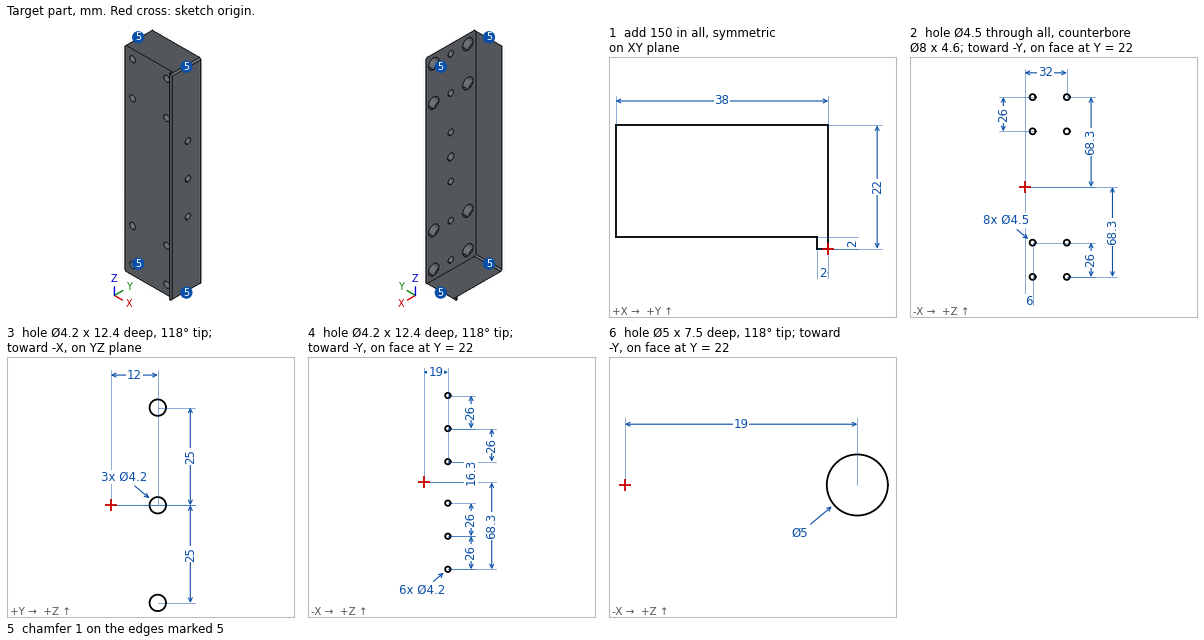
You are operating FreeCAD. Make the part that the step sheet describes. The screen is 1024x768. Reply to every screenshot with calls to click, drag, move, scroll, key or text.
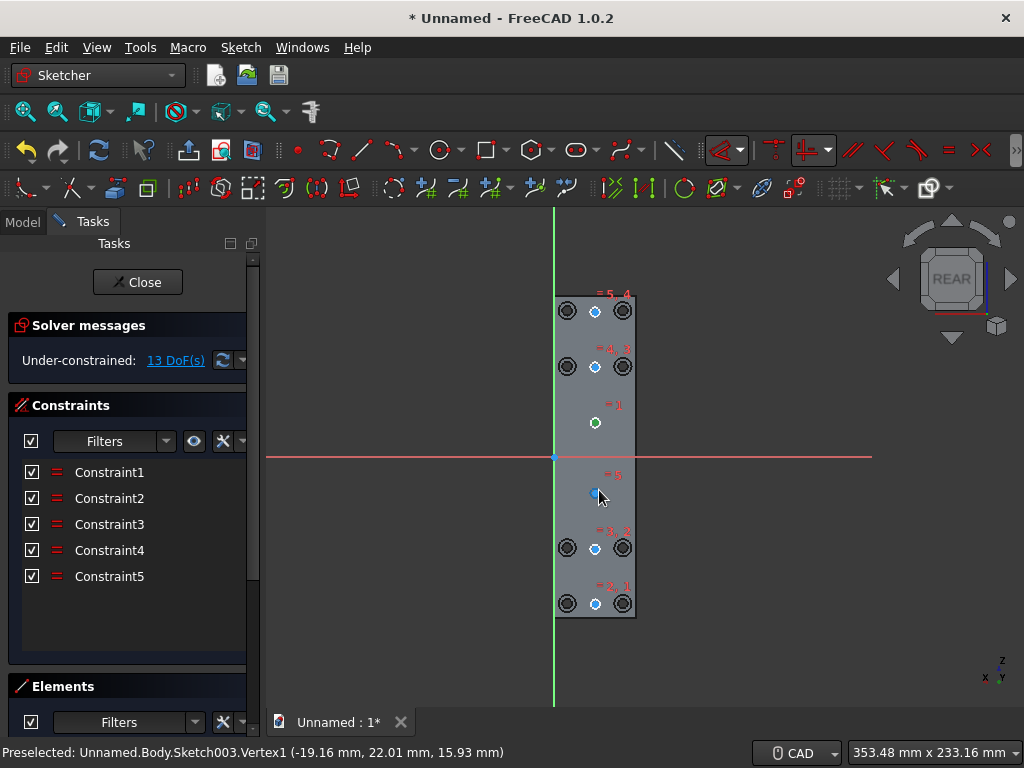
click(595, 604)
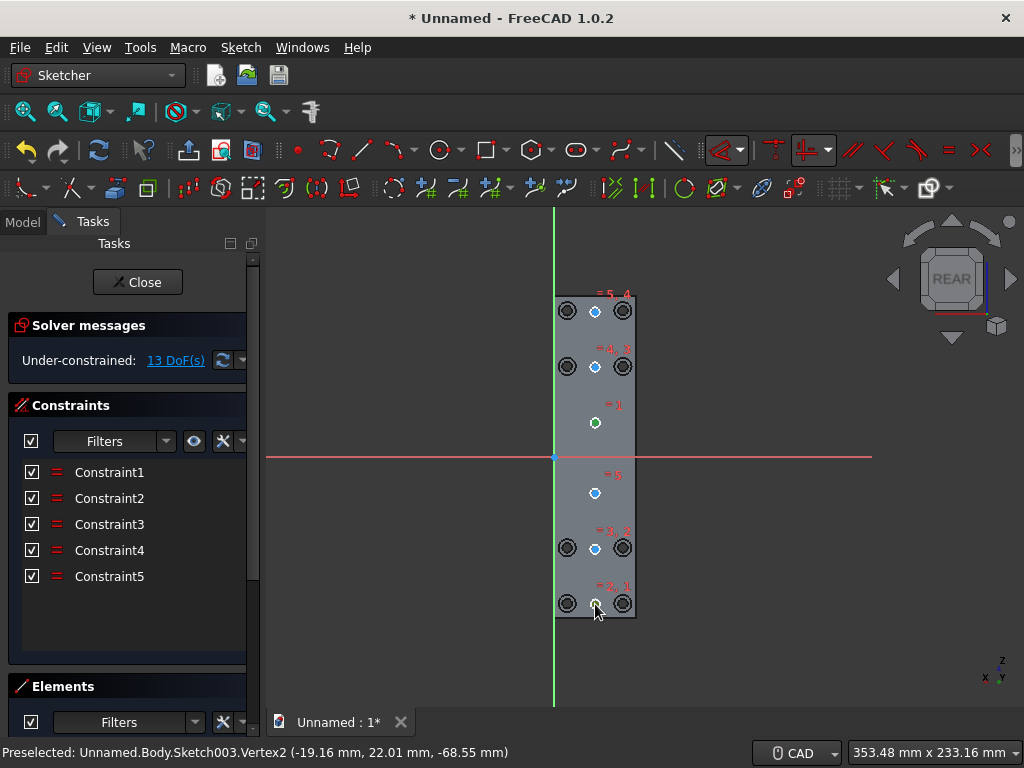
key(v)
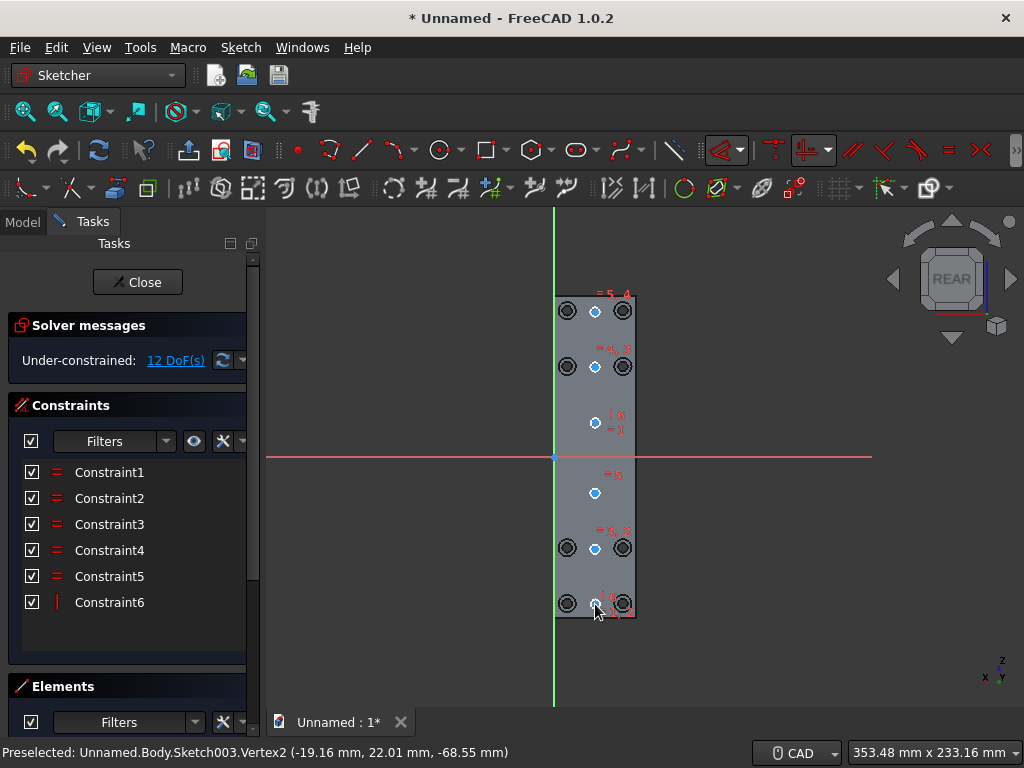
click(595, 604)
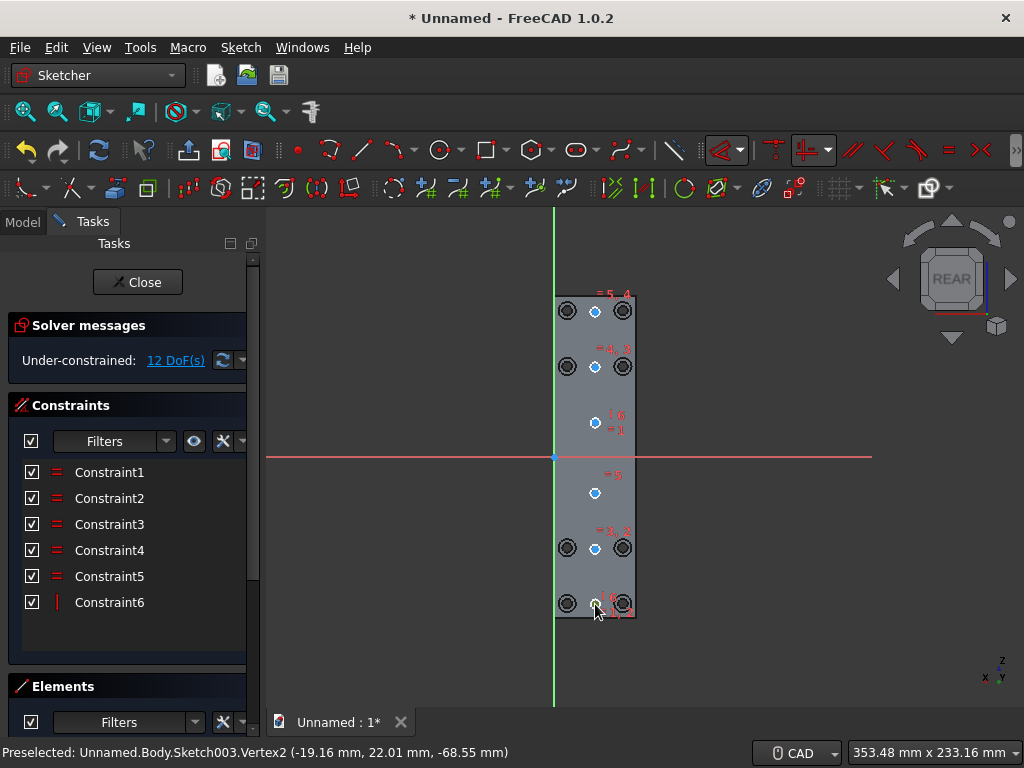
click(595, 549)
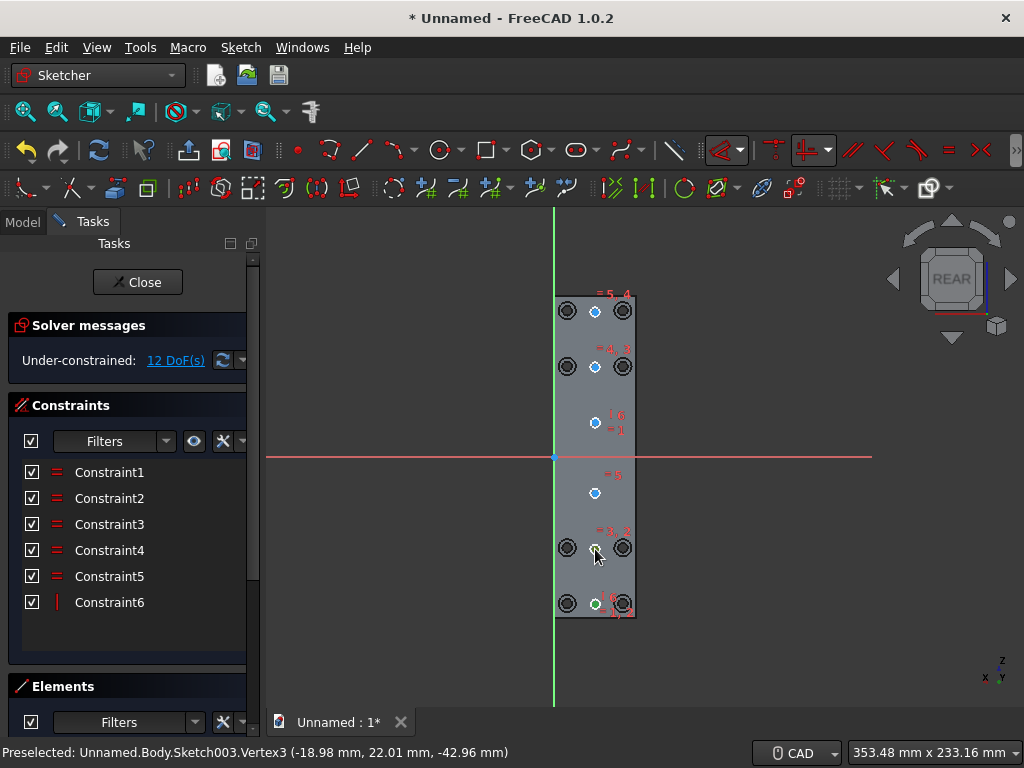
key(v)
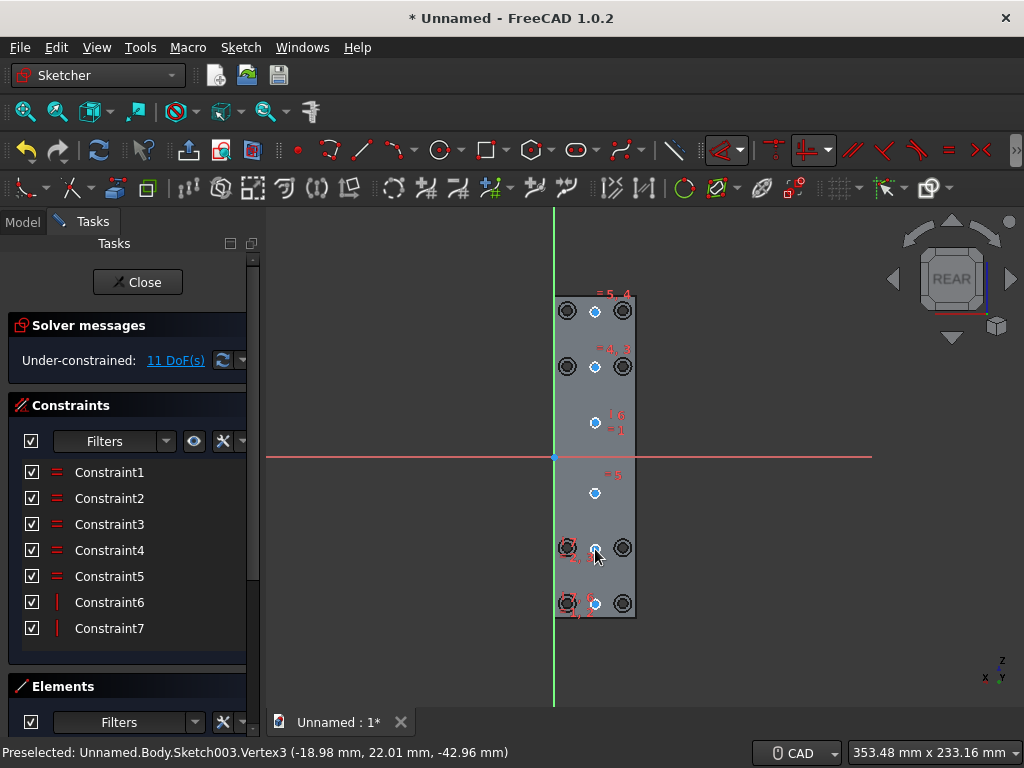
click(595, 423)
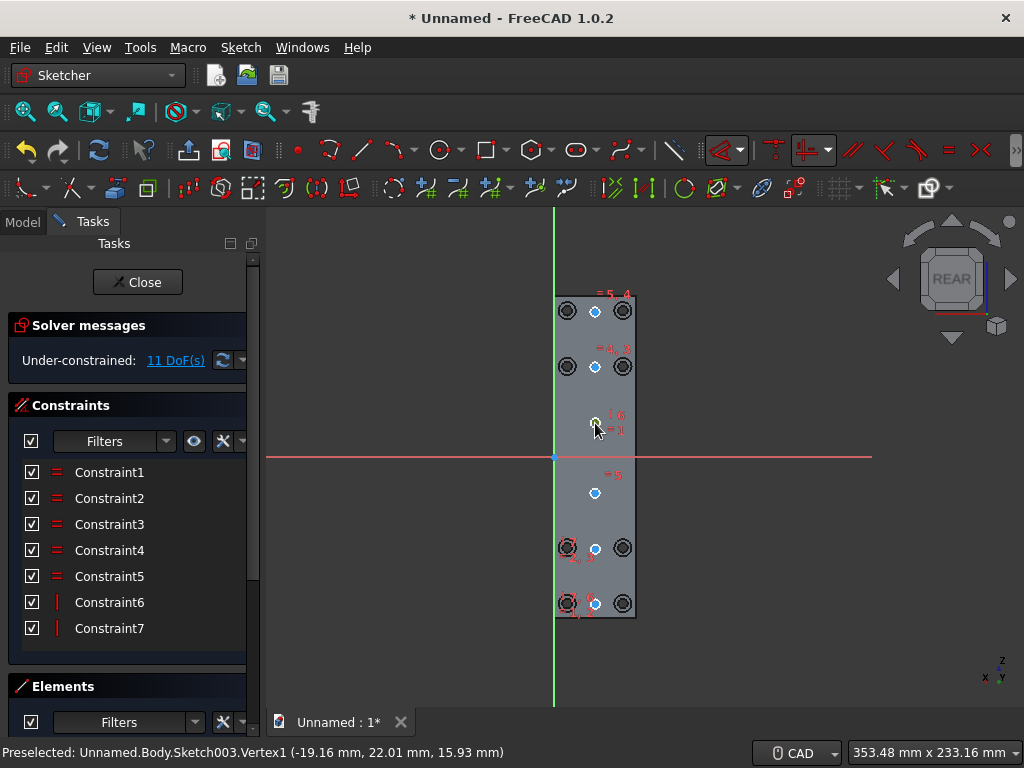
click(595, 367)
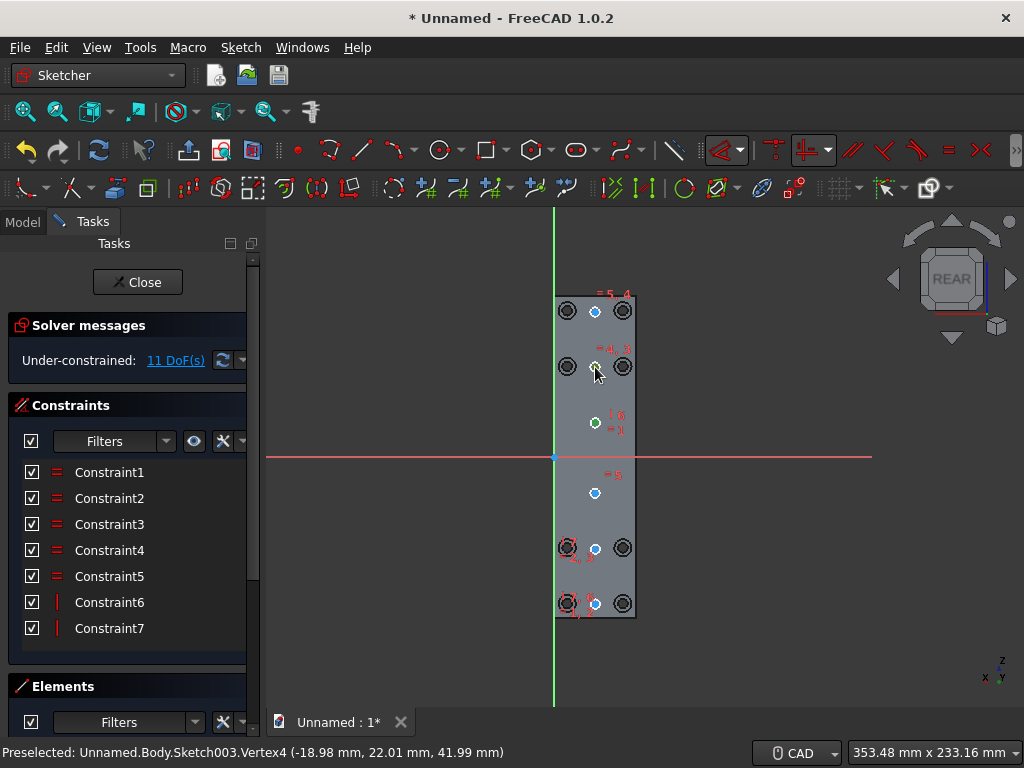
key(v)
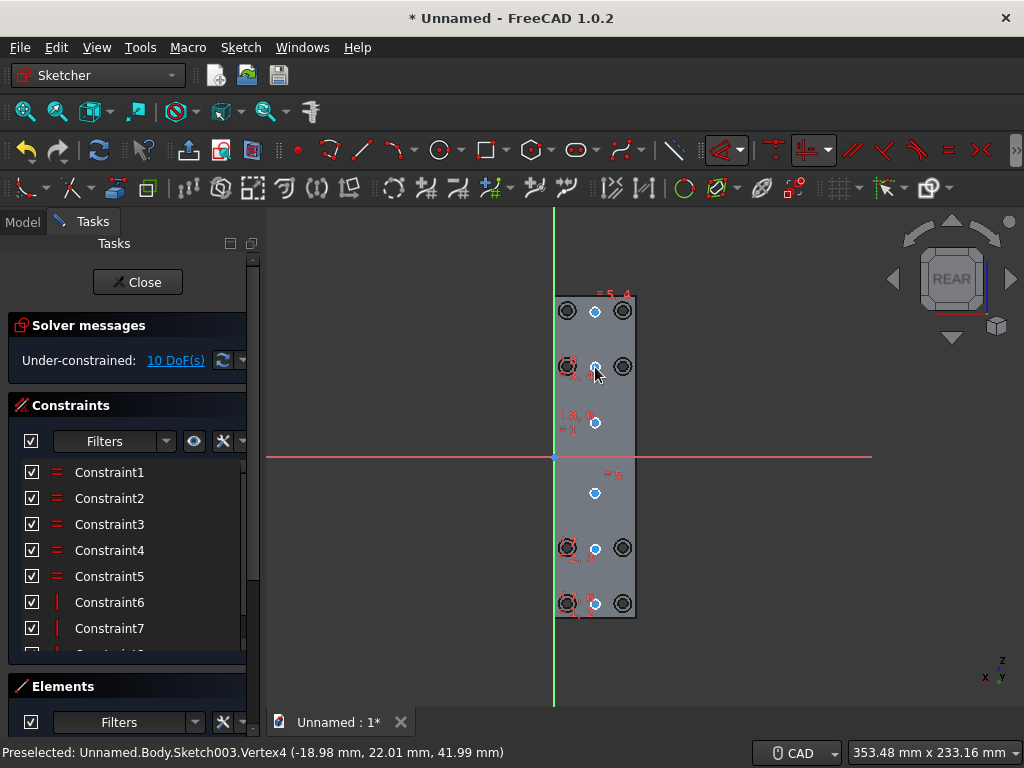
click(595, 367)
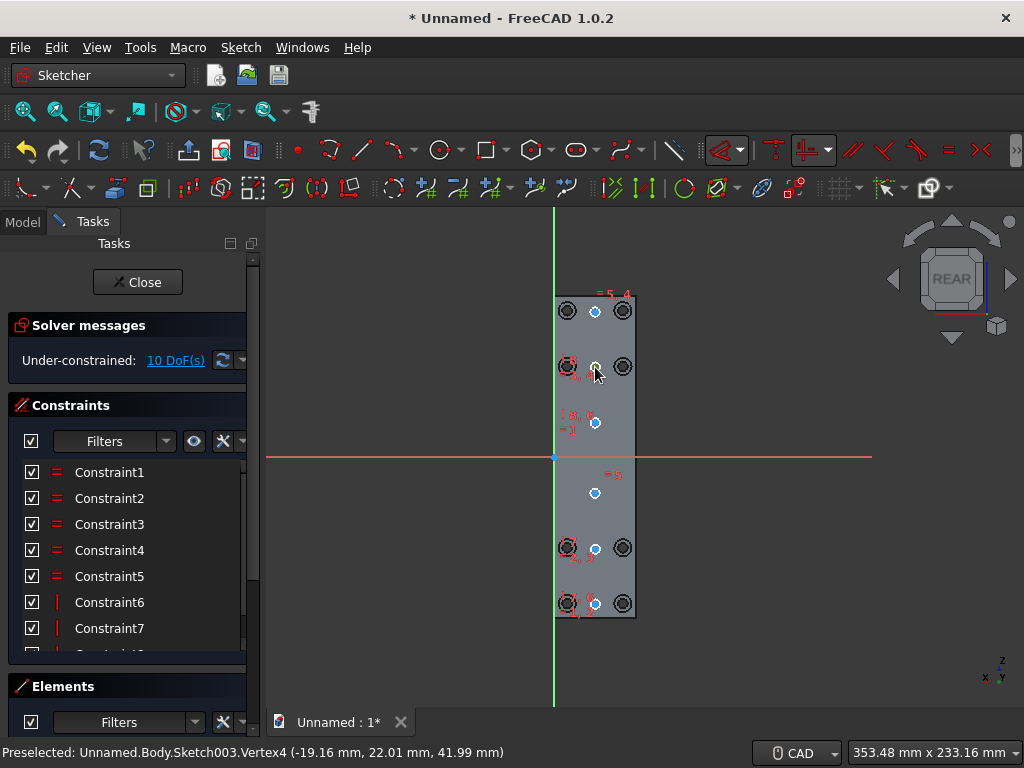
click(595, 312)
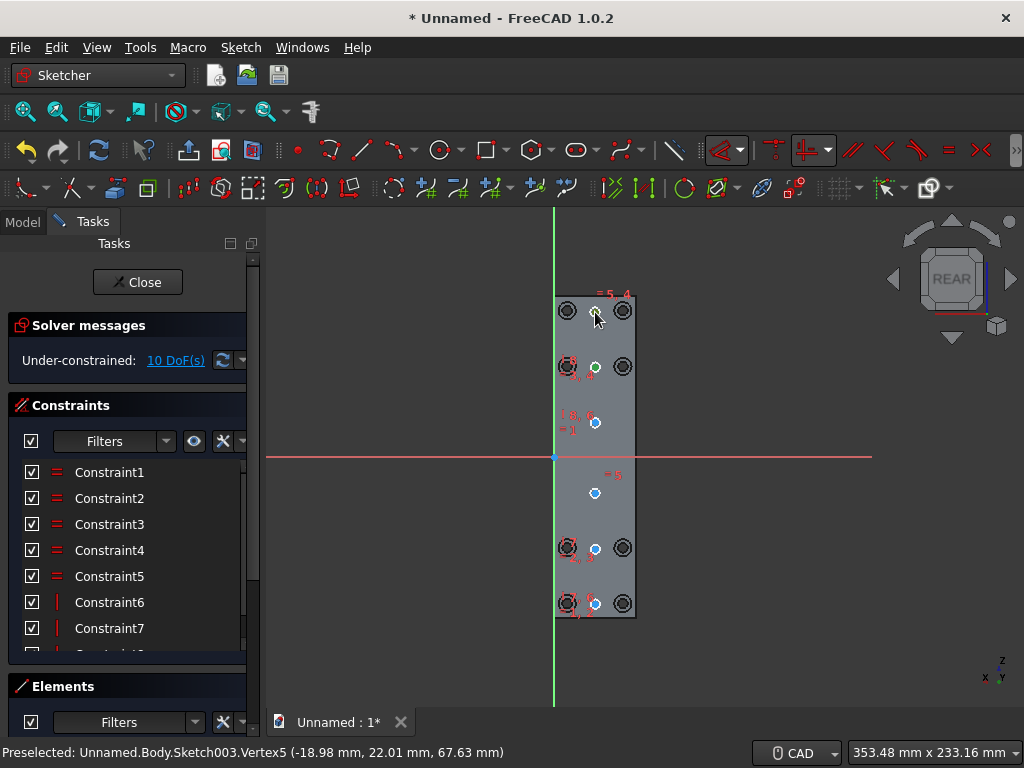
key(v)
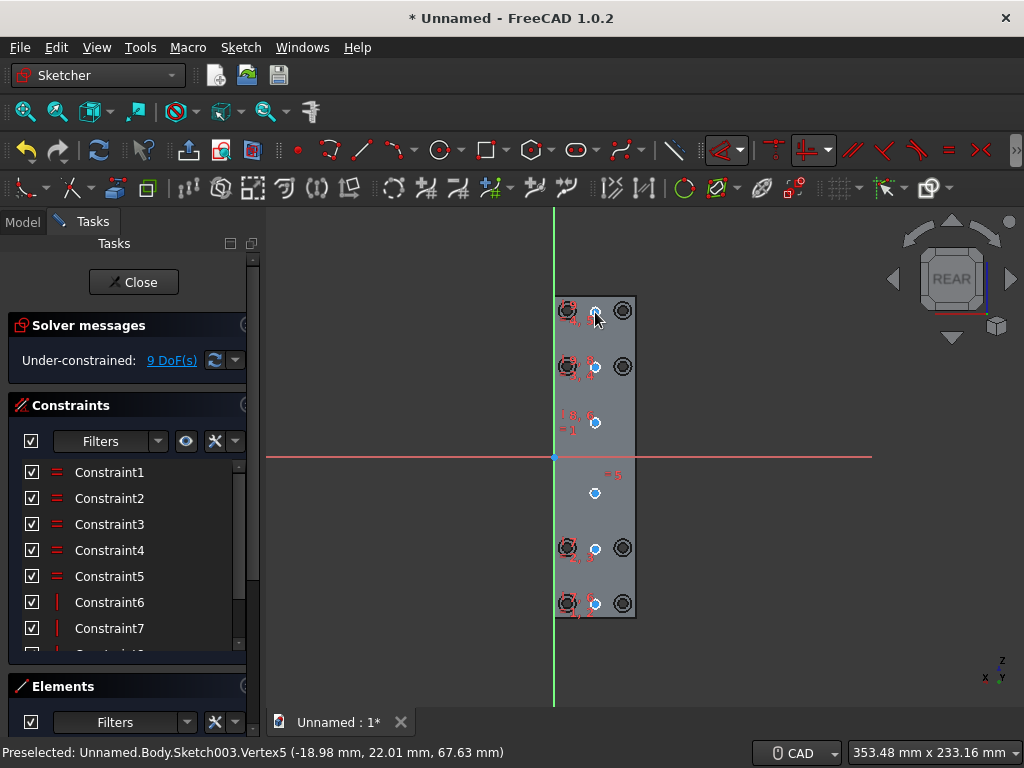
click(595, 549)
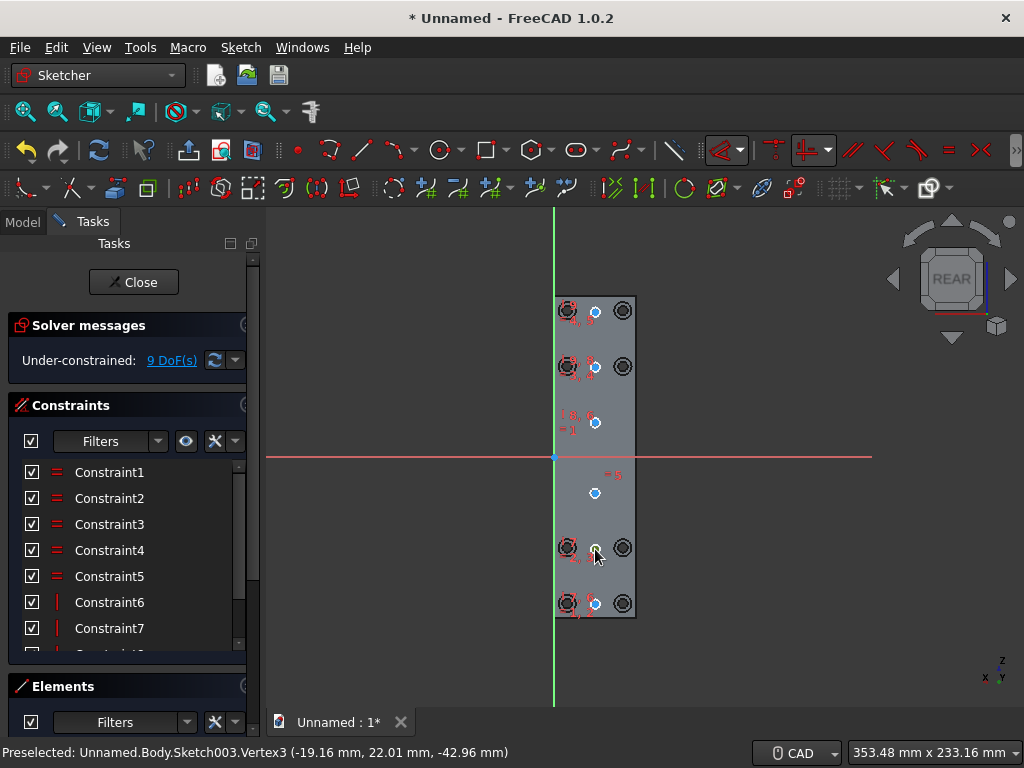
click(595, 493)